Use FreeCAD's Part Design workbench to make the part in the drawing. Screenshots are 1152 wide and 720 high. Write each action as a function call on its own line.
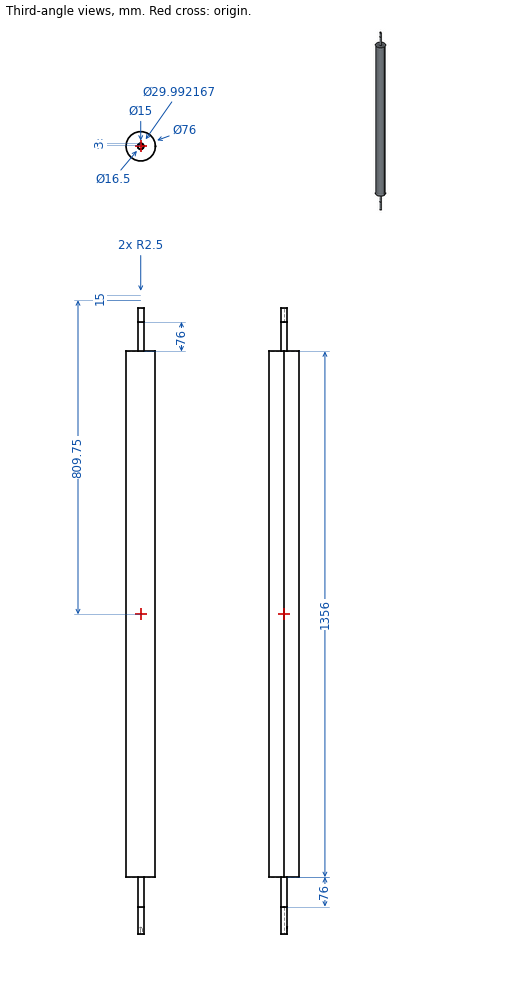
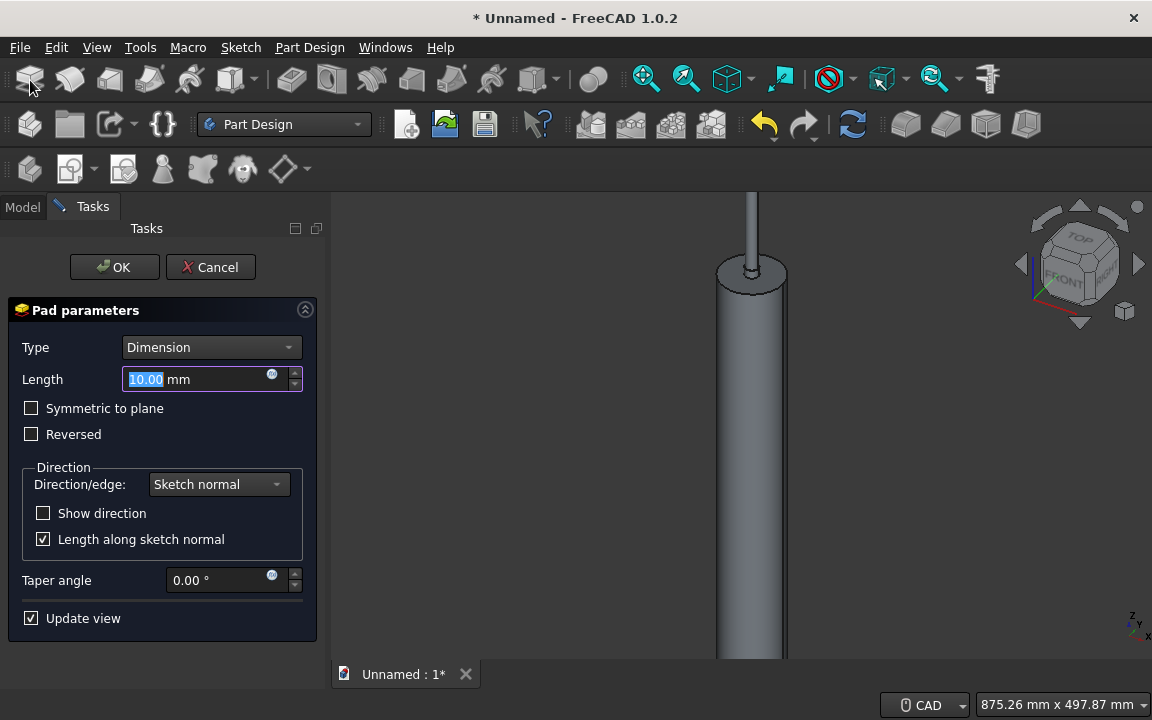
text(76)
key(Tab)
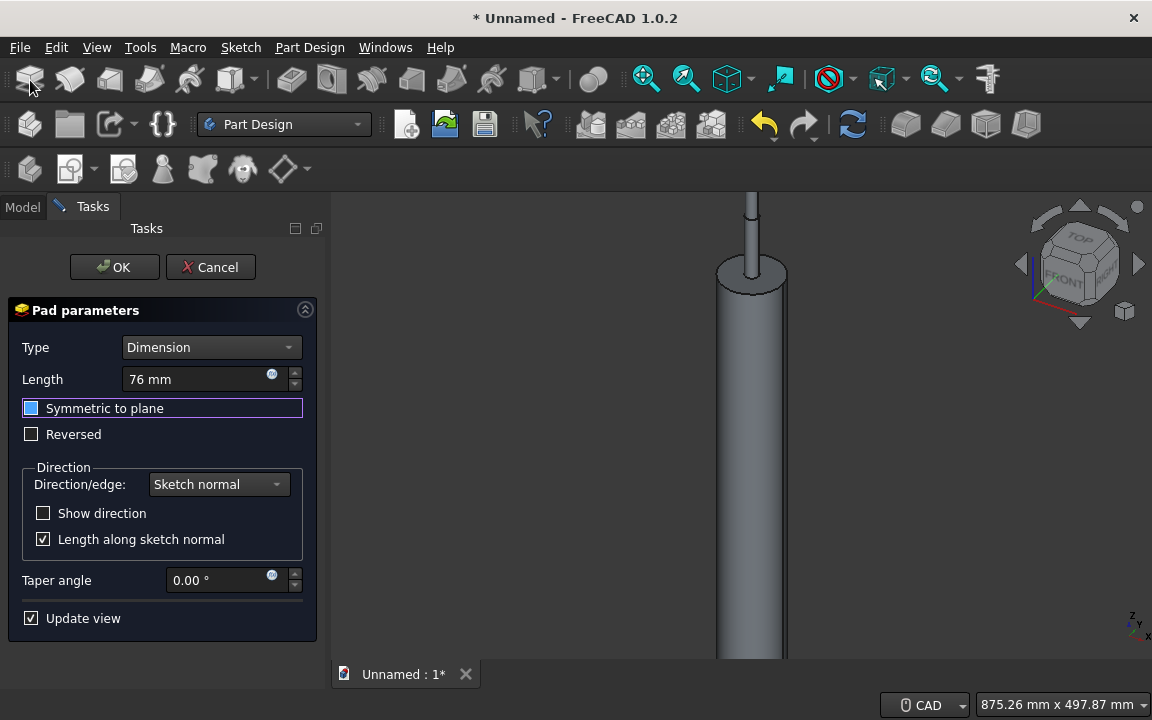
click(115, 267)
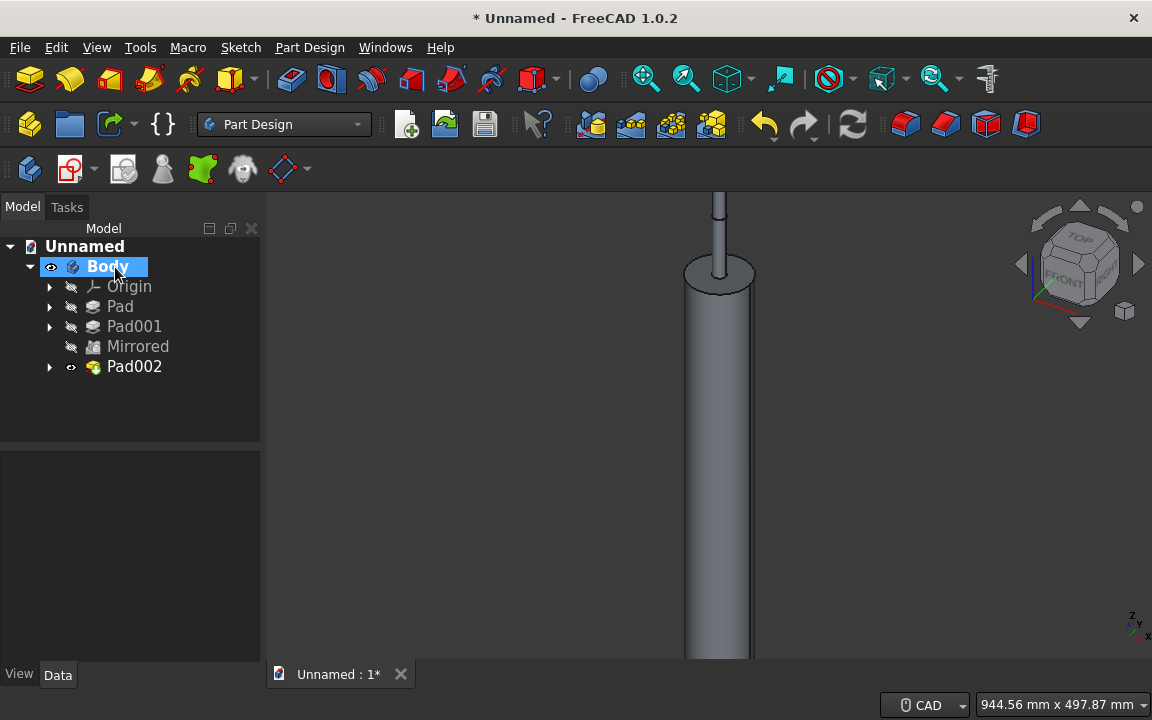
click(648, 80)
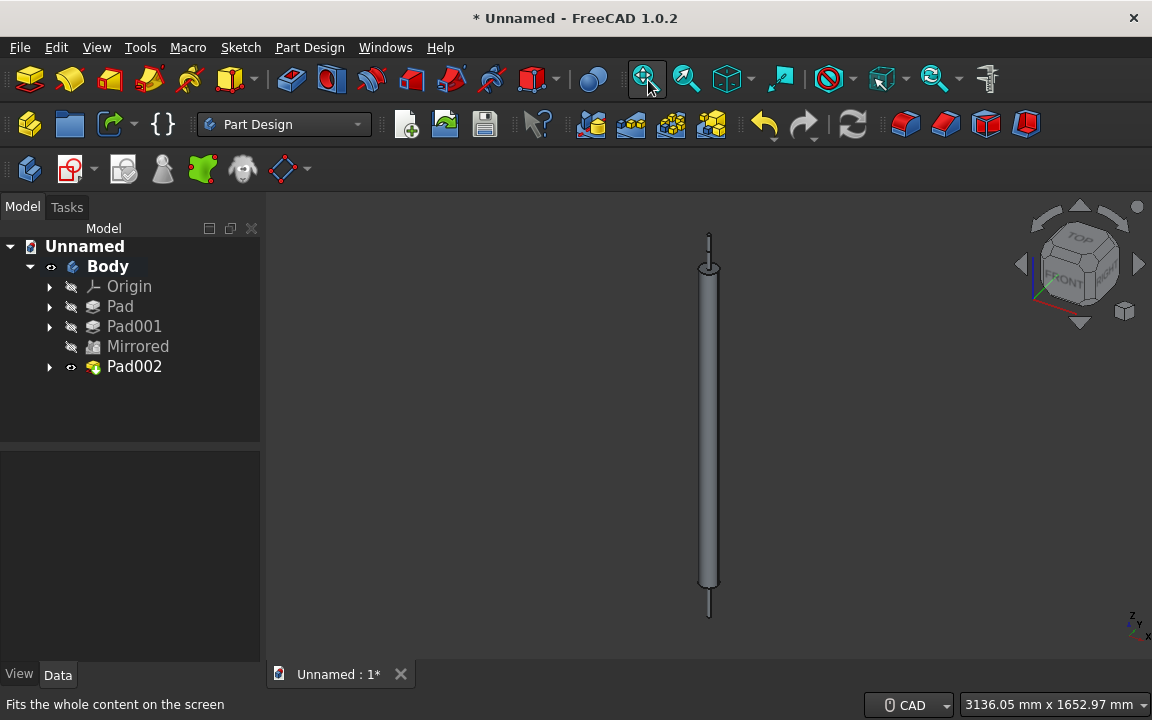
click(50, 287)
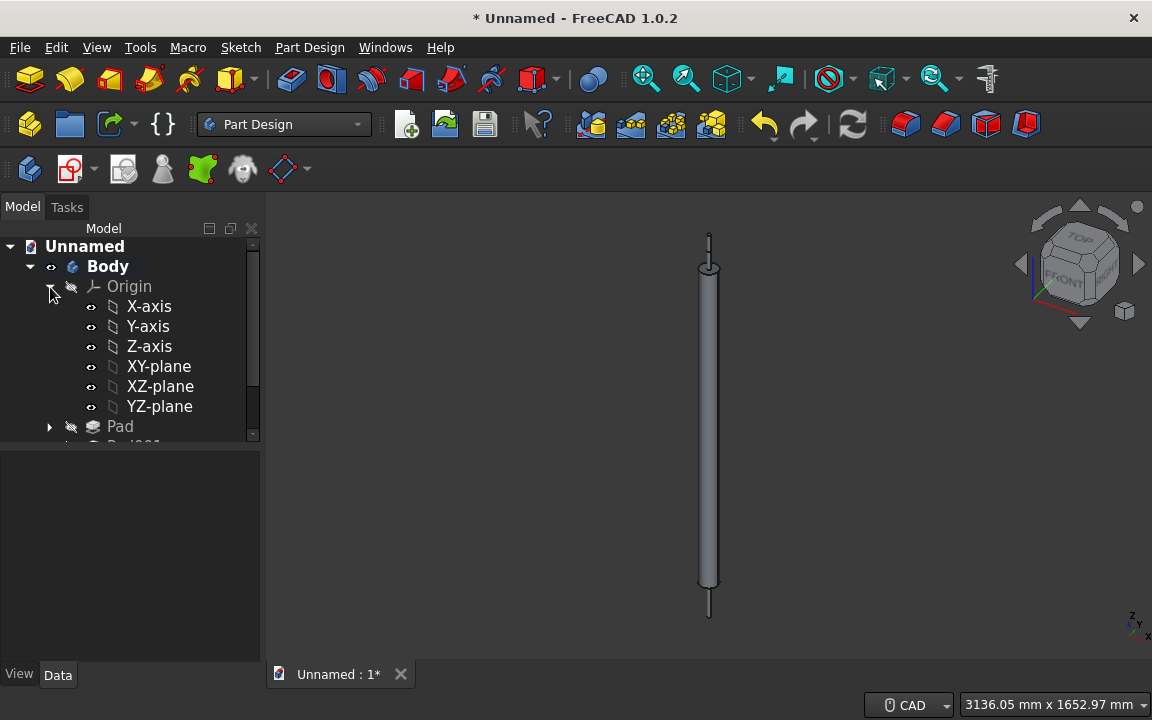
click(136, 367)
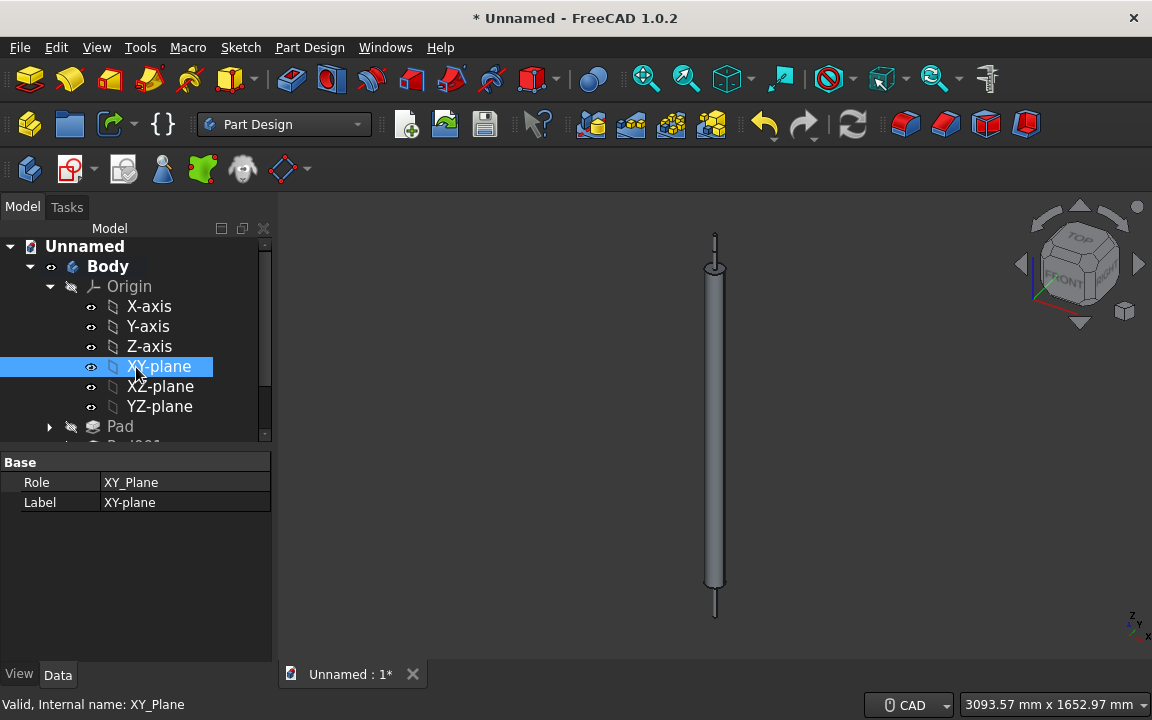
click(284, 170)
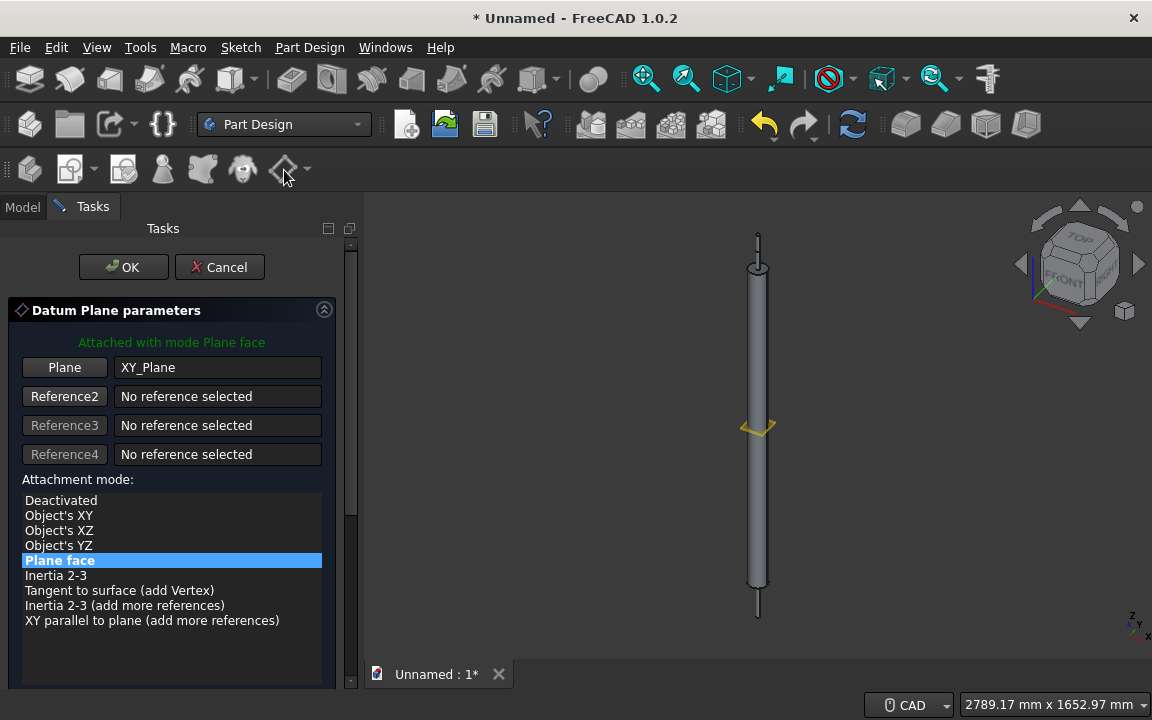
scroll(351, 463, down, 3)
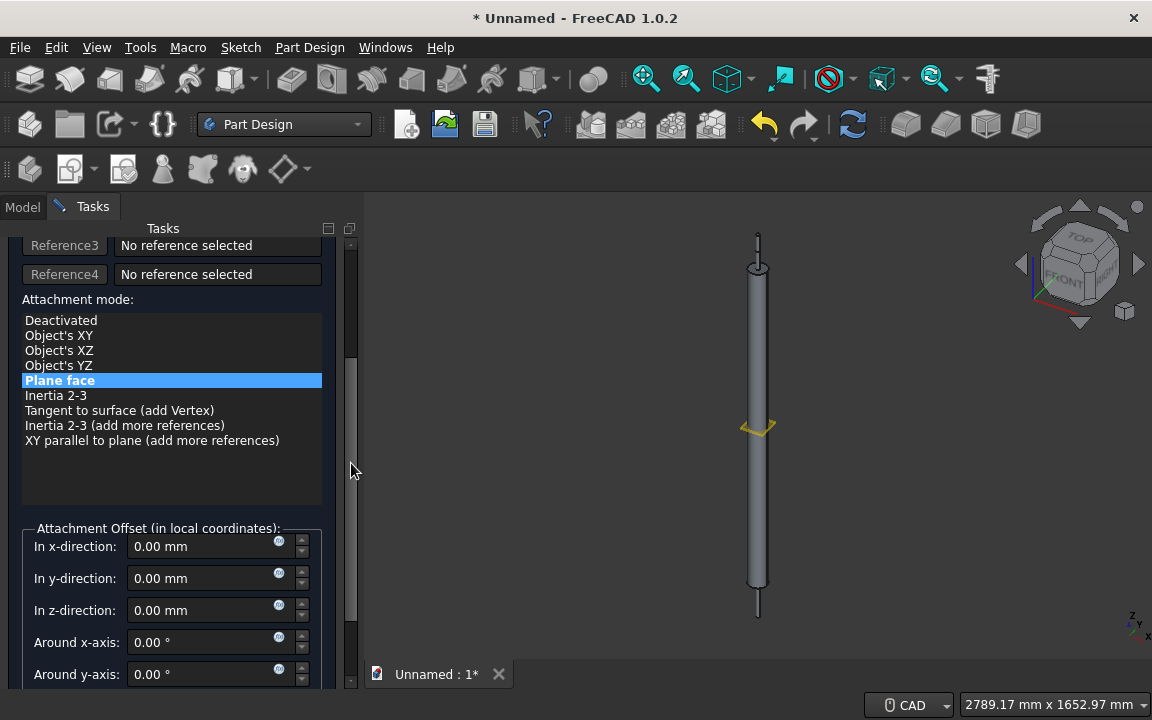
triple_click(210, 610)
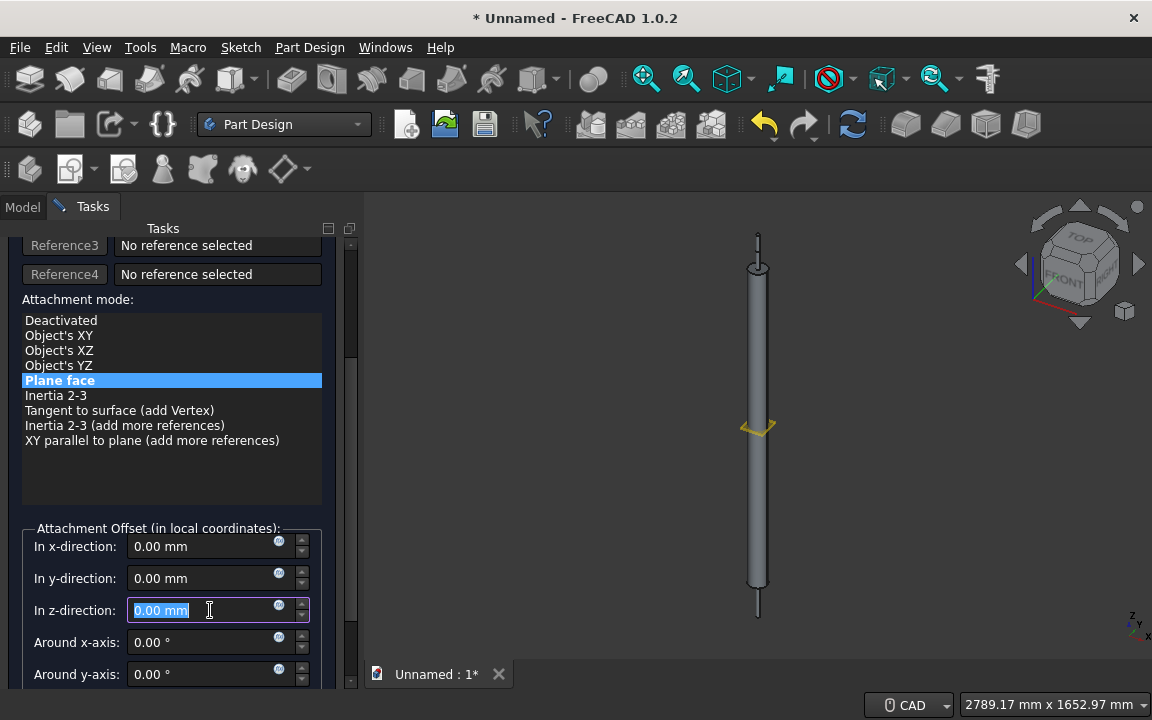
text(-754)
key(Tab)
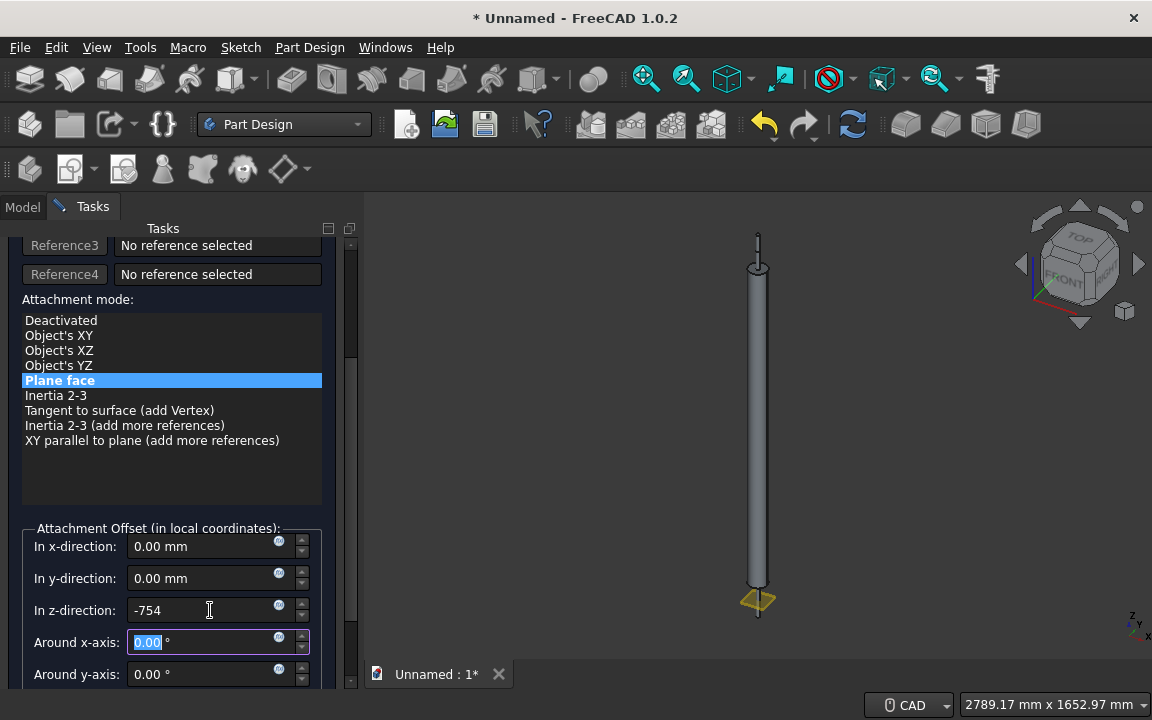
scroll(351, 463, up, 4)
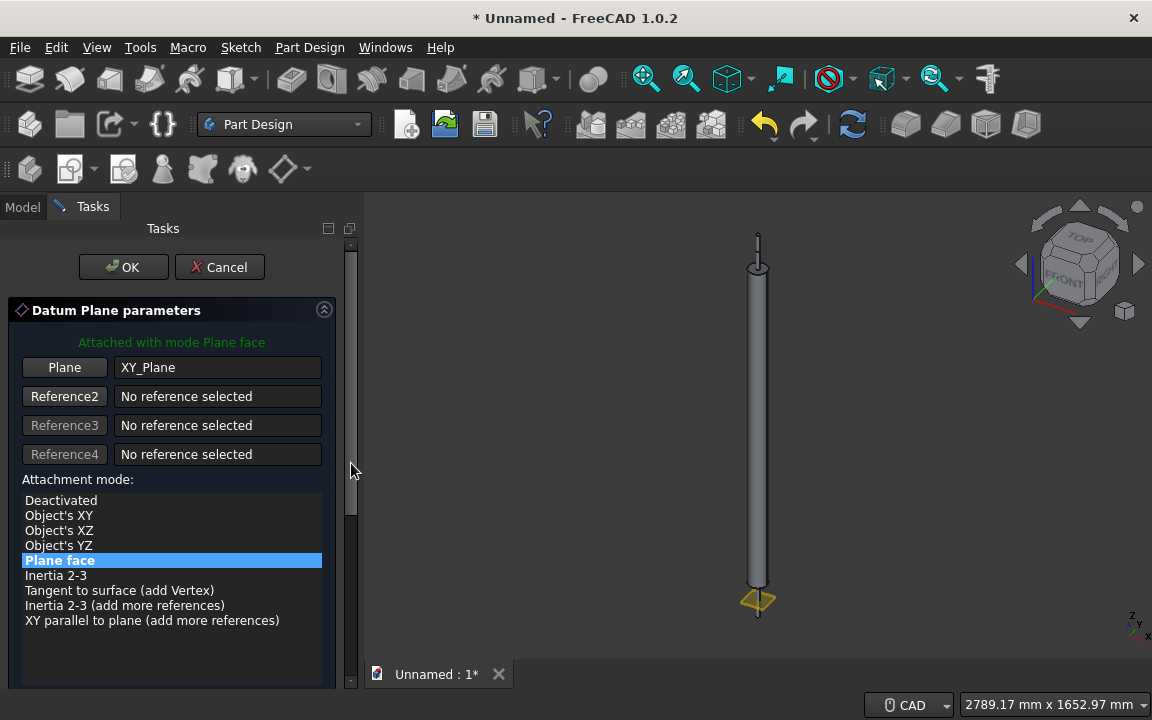
click(124, 267)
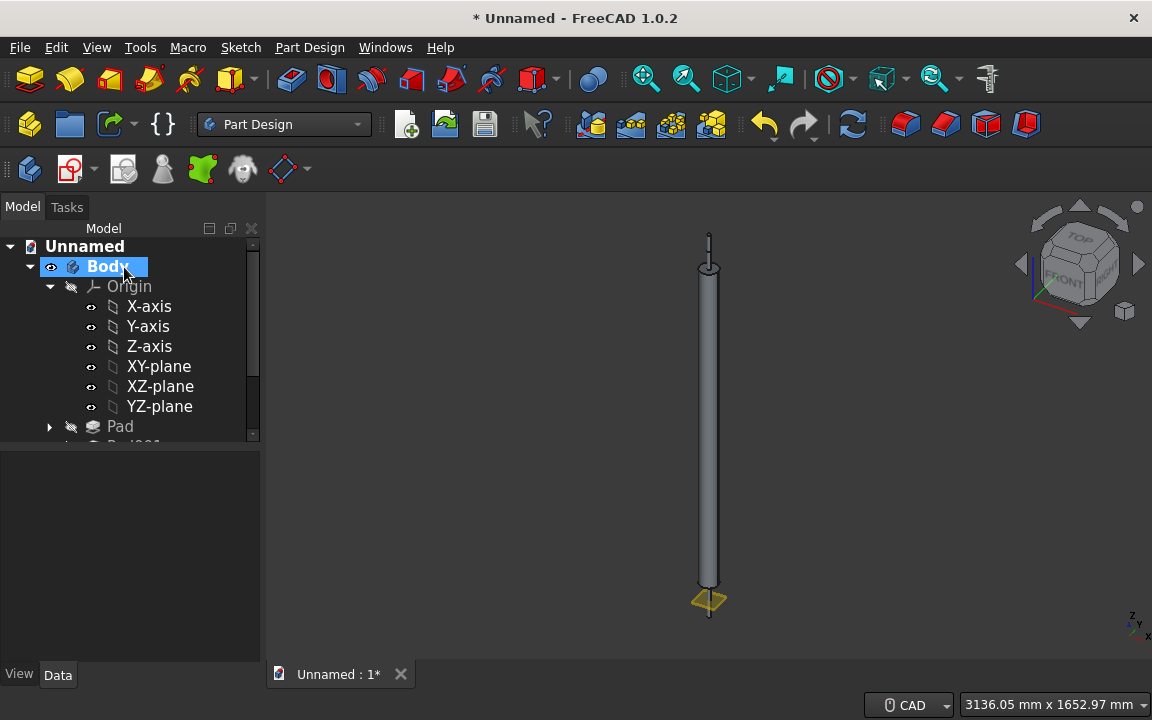
scroll(100, 342, down, 3)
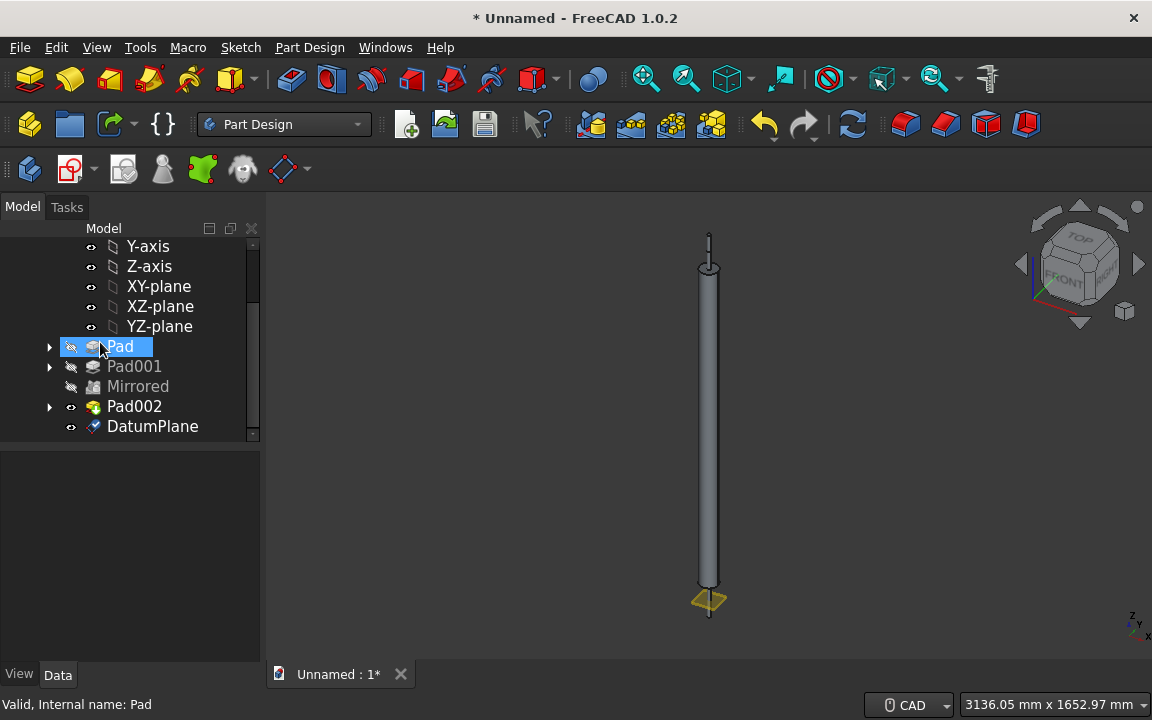
click(116, 427)